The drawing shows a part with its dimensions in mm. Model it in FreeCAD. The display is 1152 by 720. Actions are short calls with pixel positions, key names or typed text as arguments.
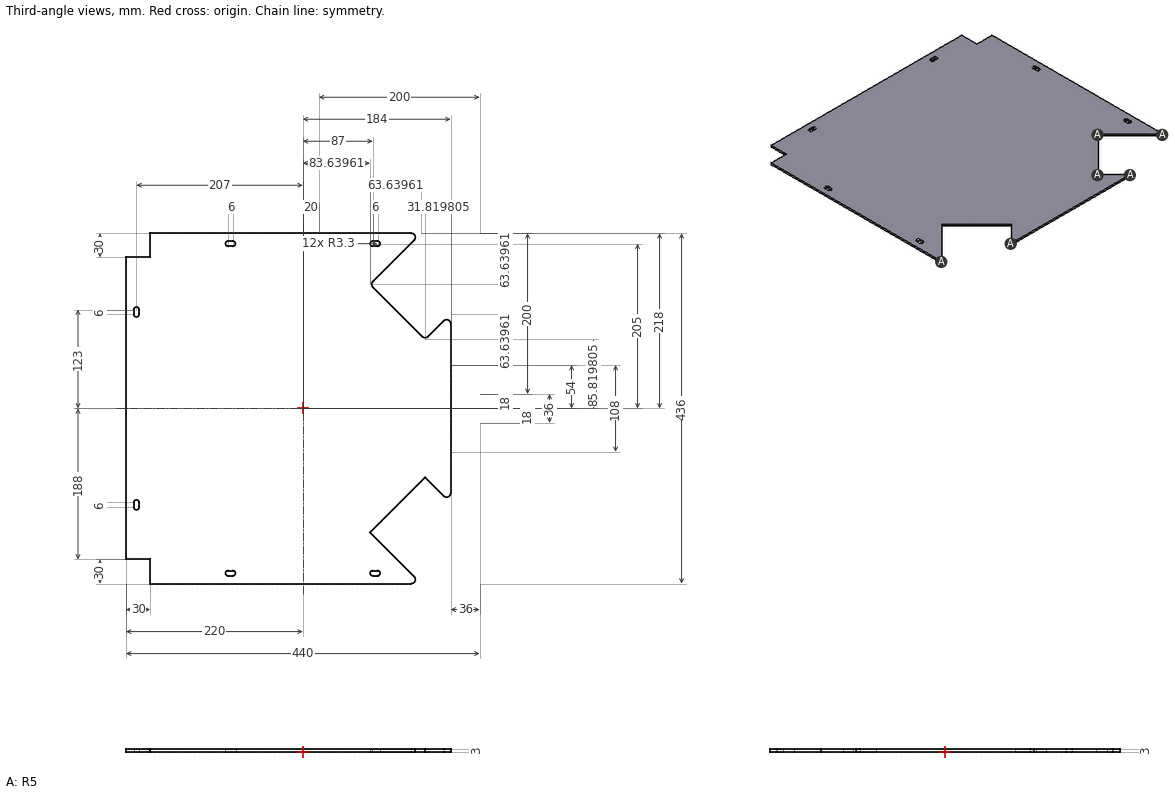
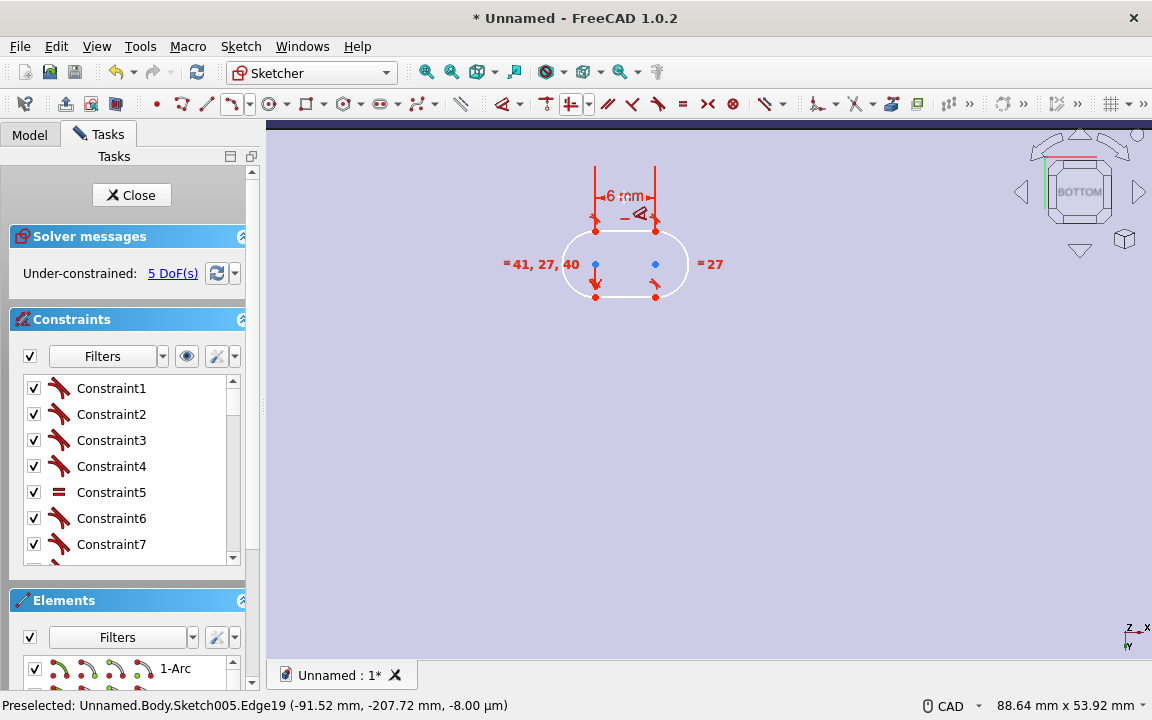
scroll(615, 236, down, 13)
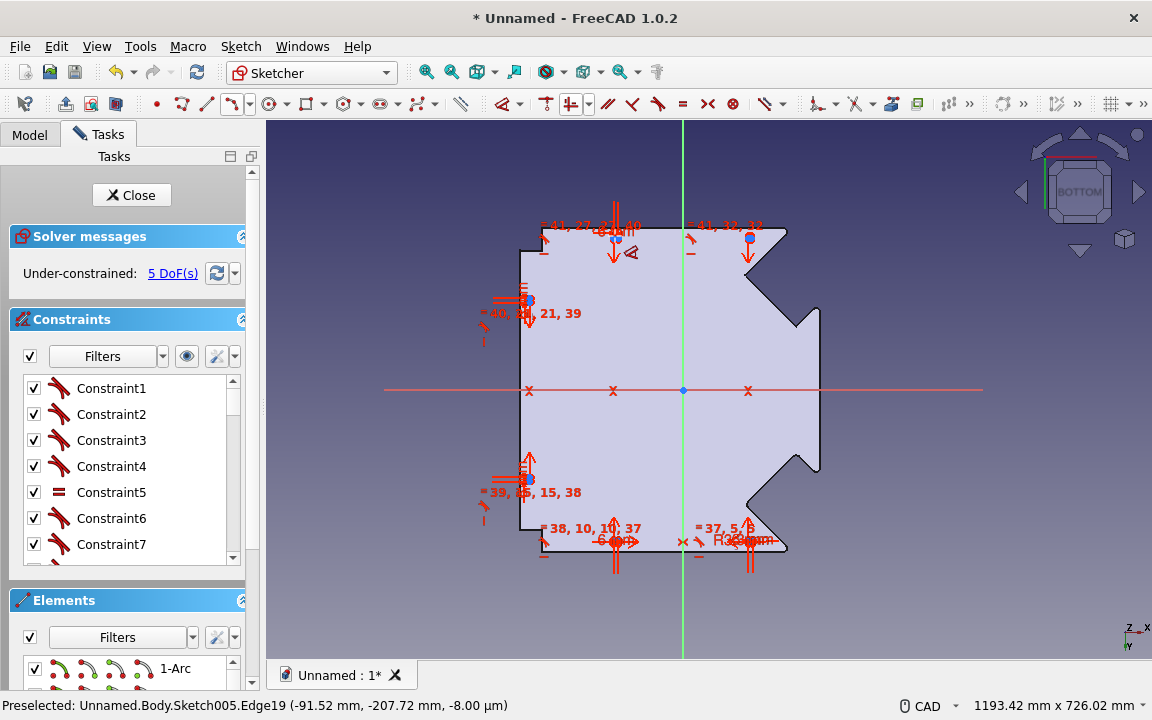
scroll(749, 236, up, 13)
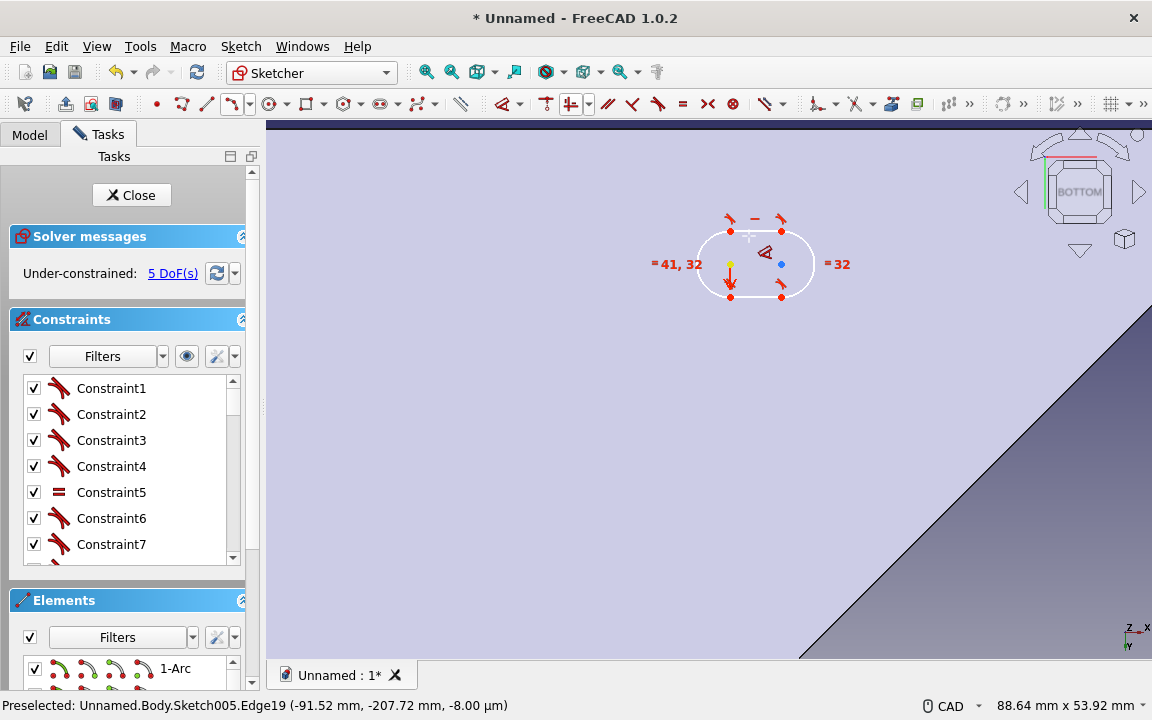
click(746, 231)
click(756, 197)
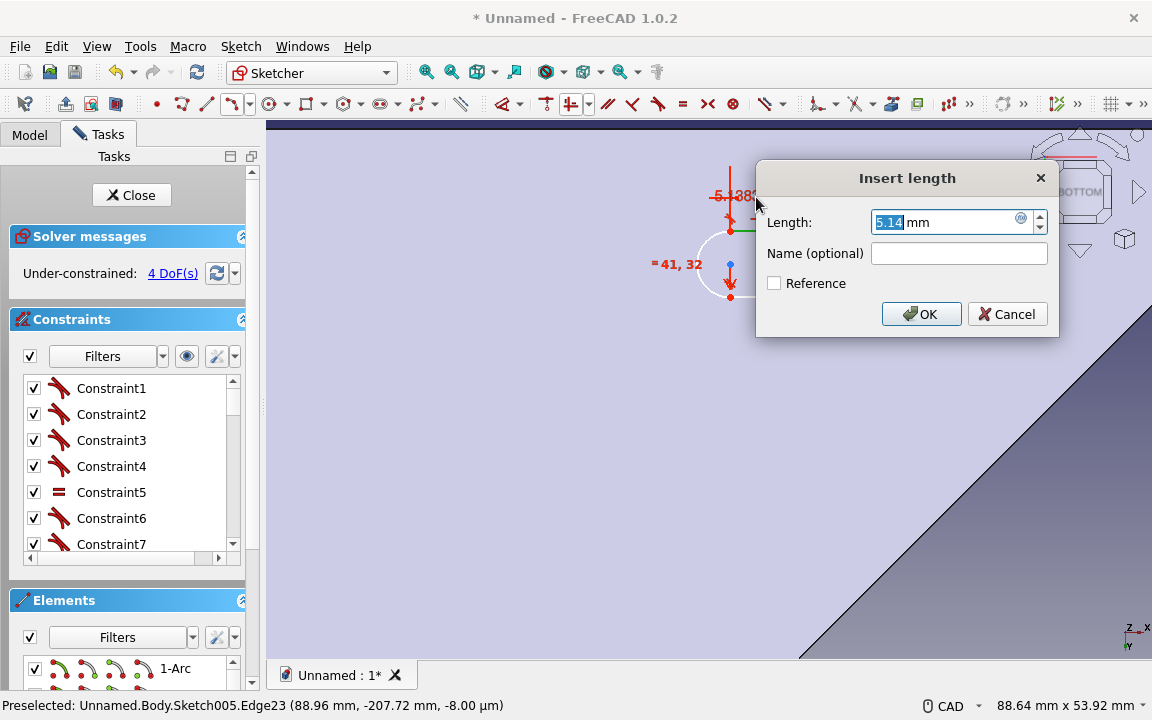
text(6)
key(Return)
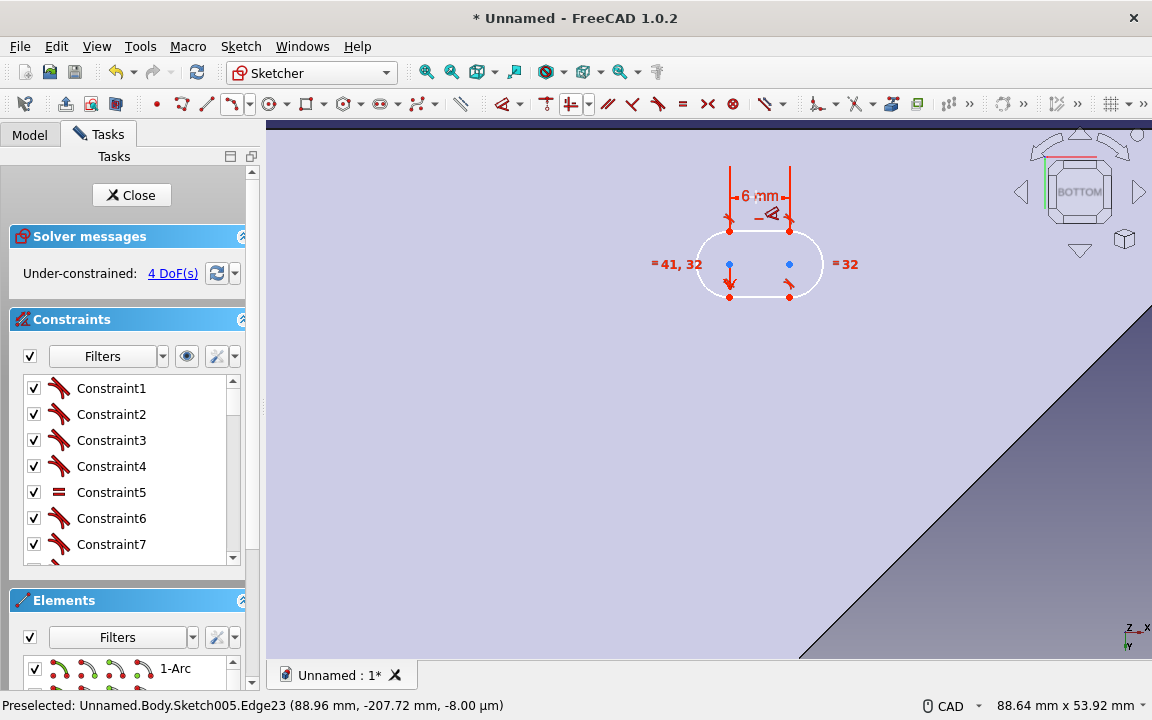
scroll(749, 236, down, 13)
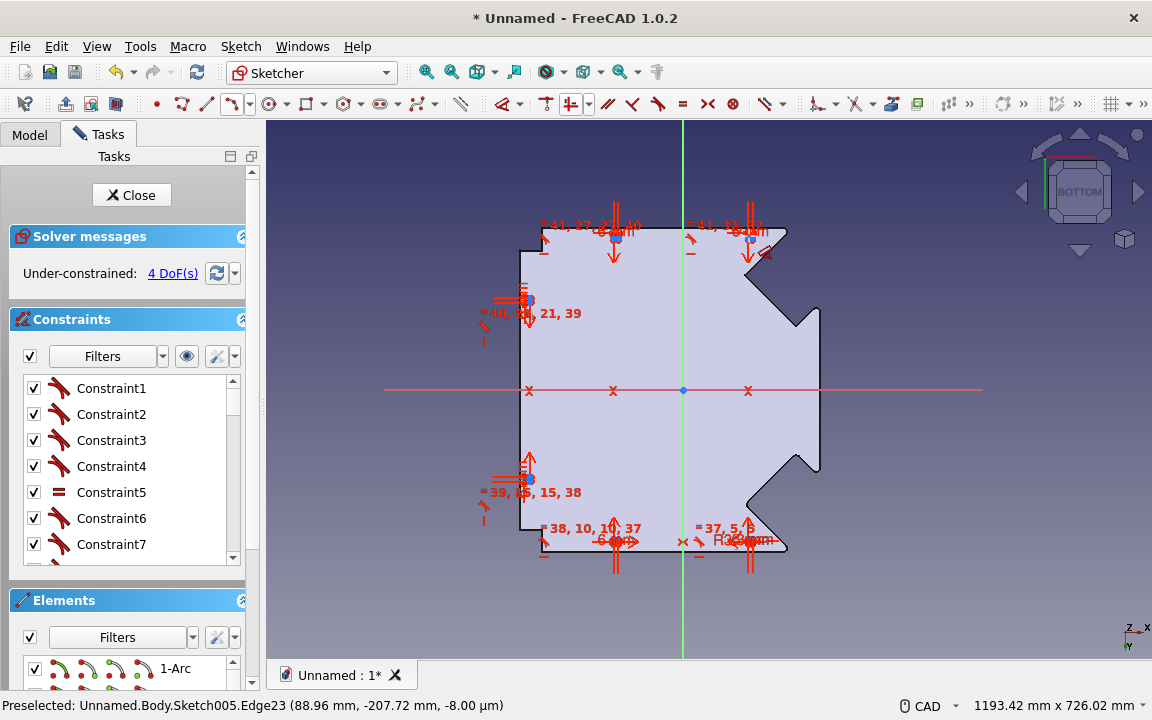
scroll(748, 539, up, 9)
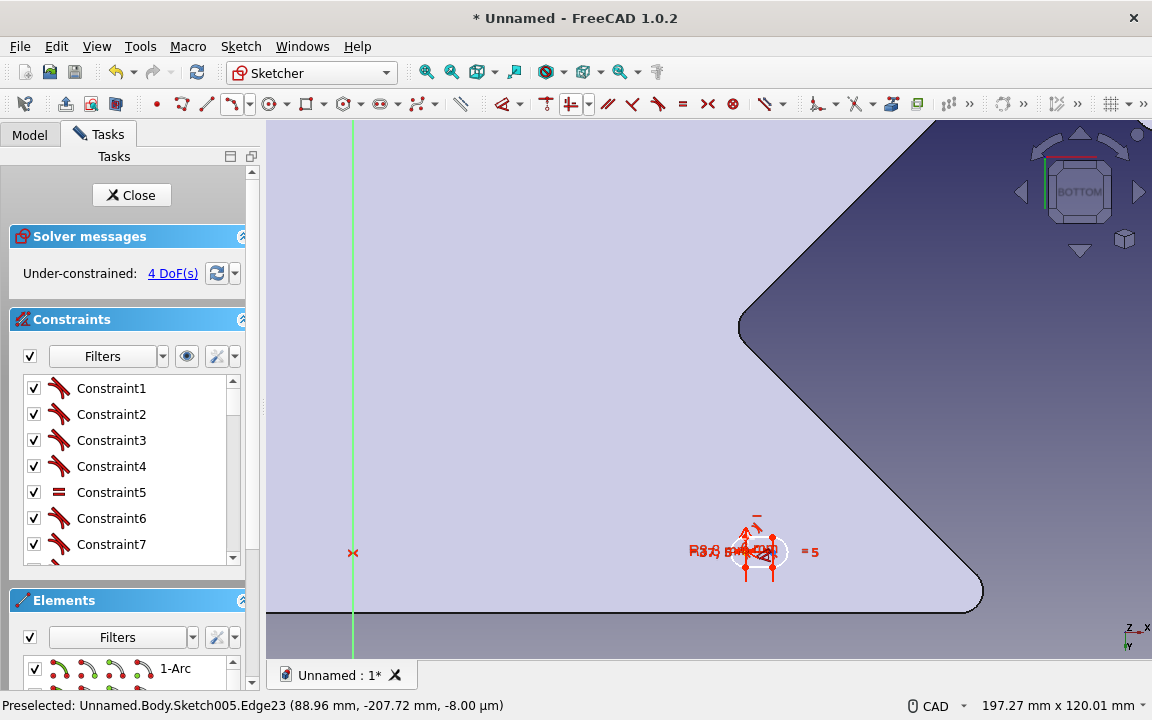
click(746, 537)
click(550, 571)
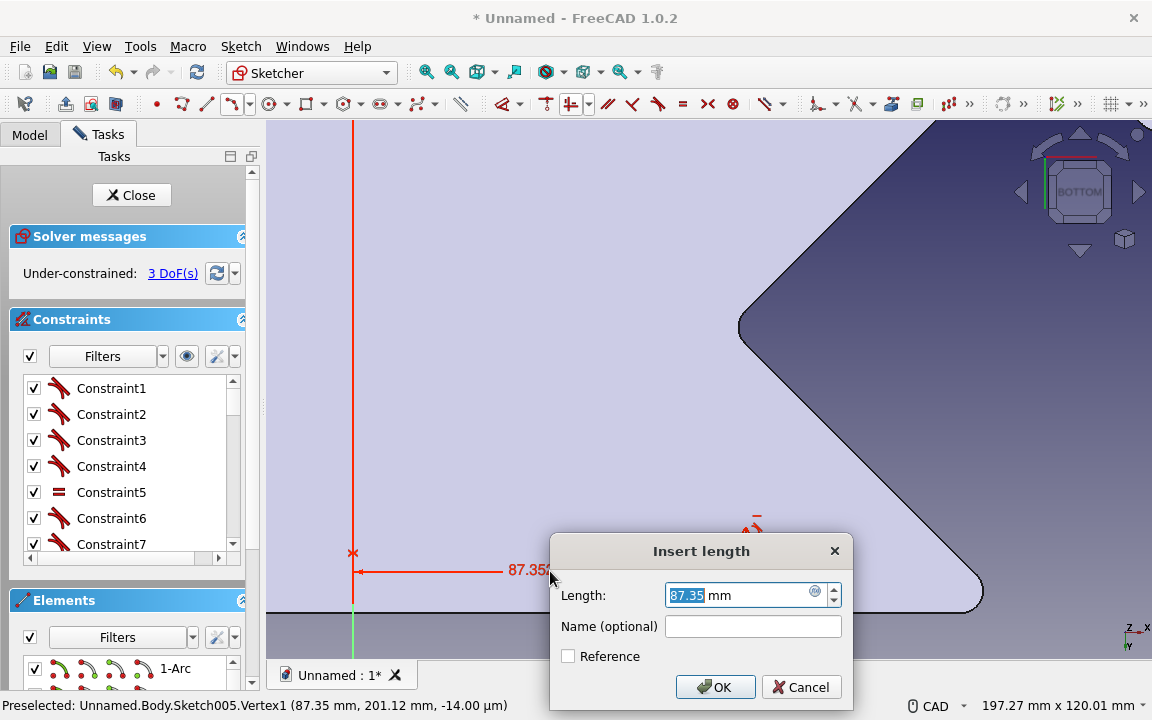
text(87)
key(Return)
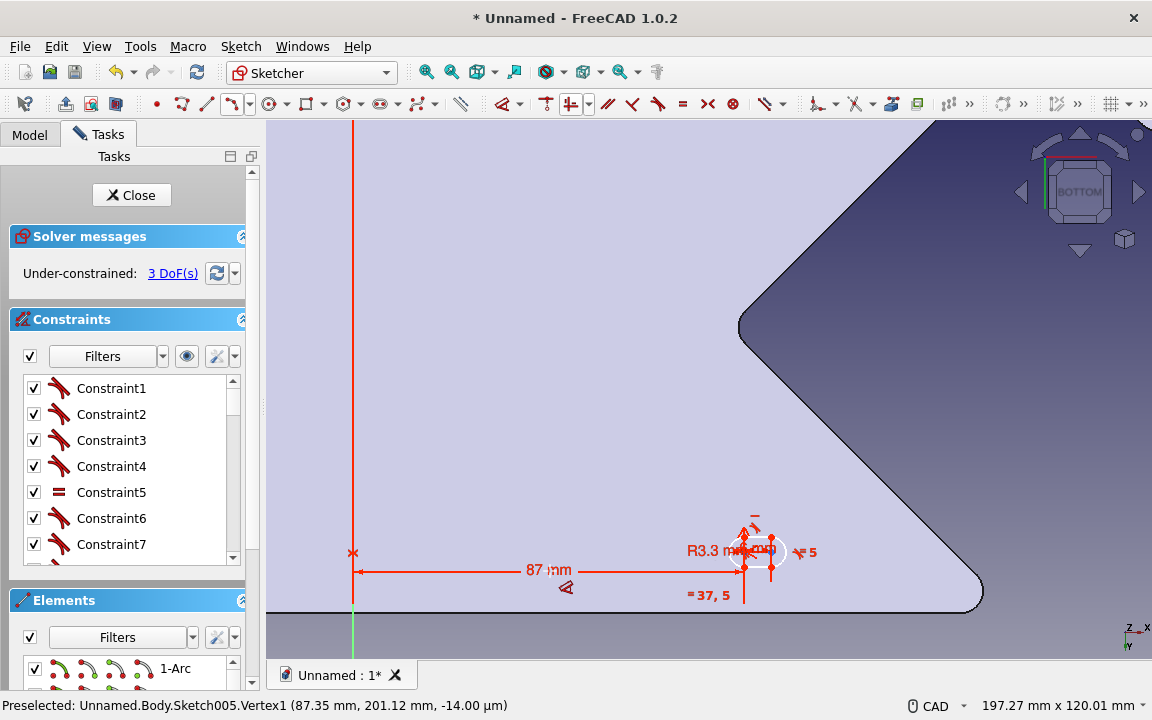
scroll(748, 539, down, 9)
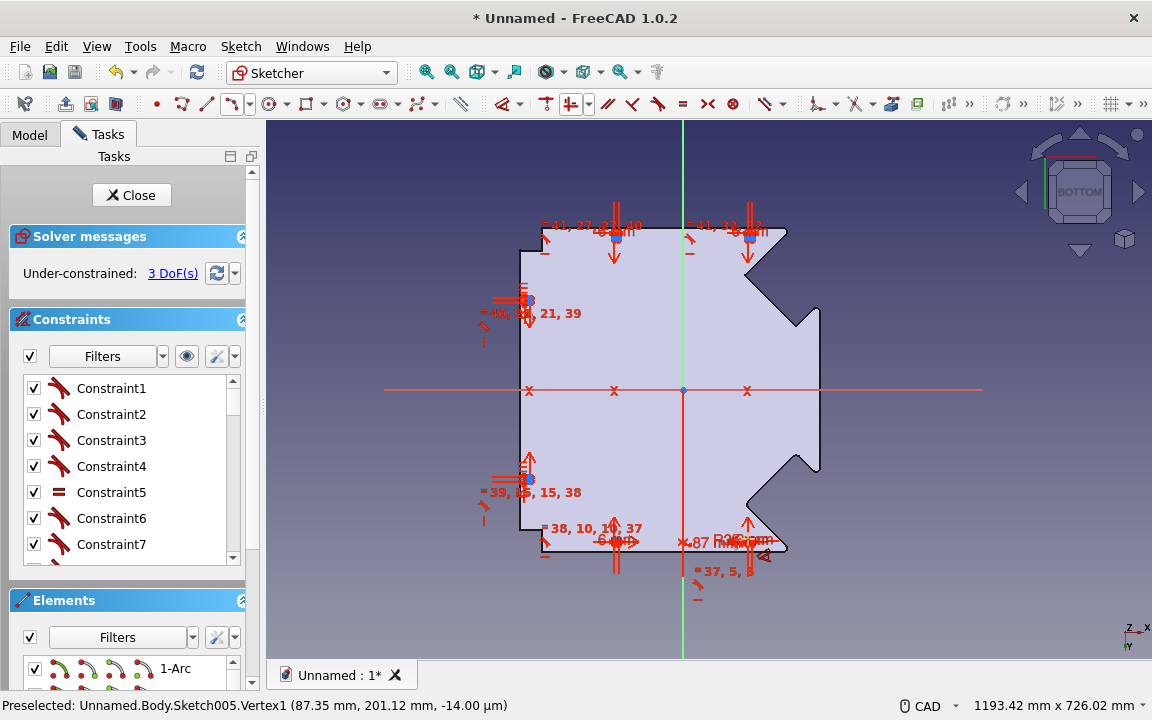
scroll(527, 482, up, 9)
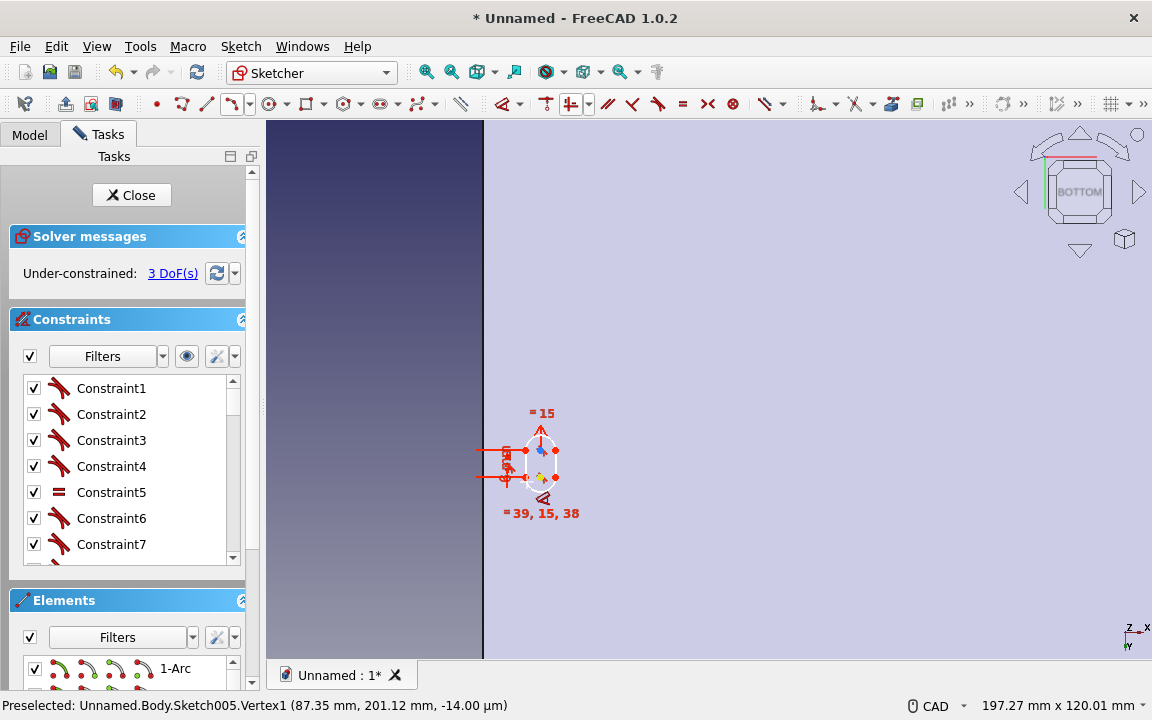
click(526, 477)
click(492, 313)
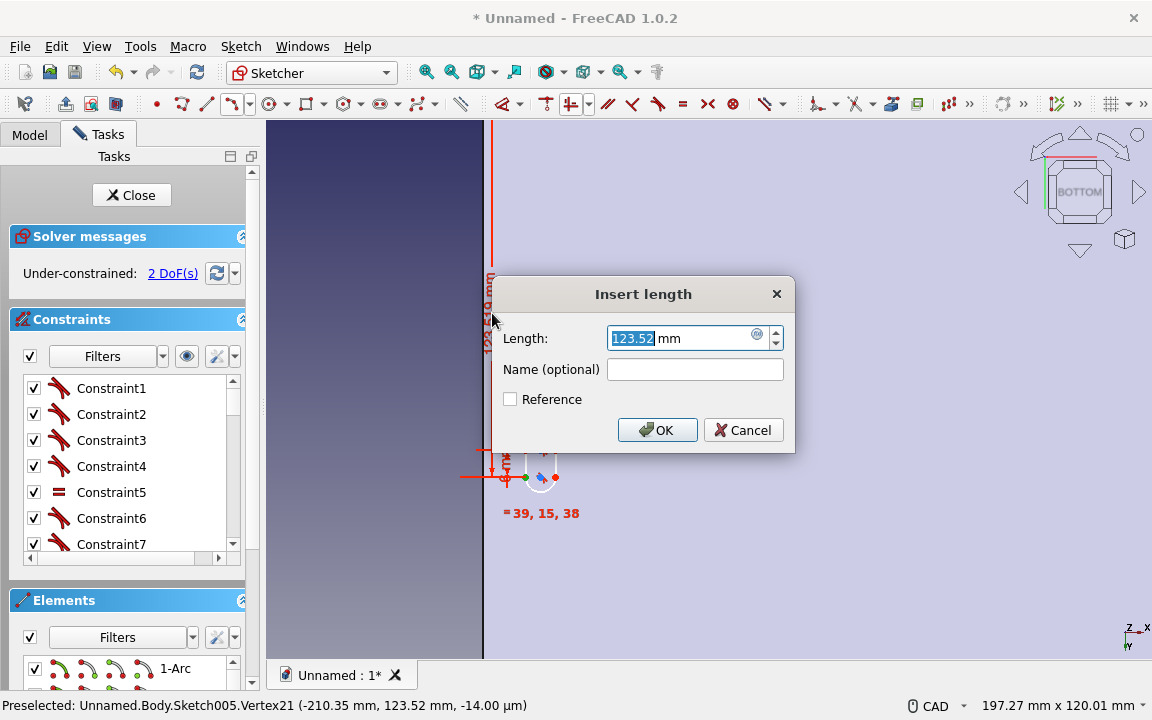
text(123)
key(Return)